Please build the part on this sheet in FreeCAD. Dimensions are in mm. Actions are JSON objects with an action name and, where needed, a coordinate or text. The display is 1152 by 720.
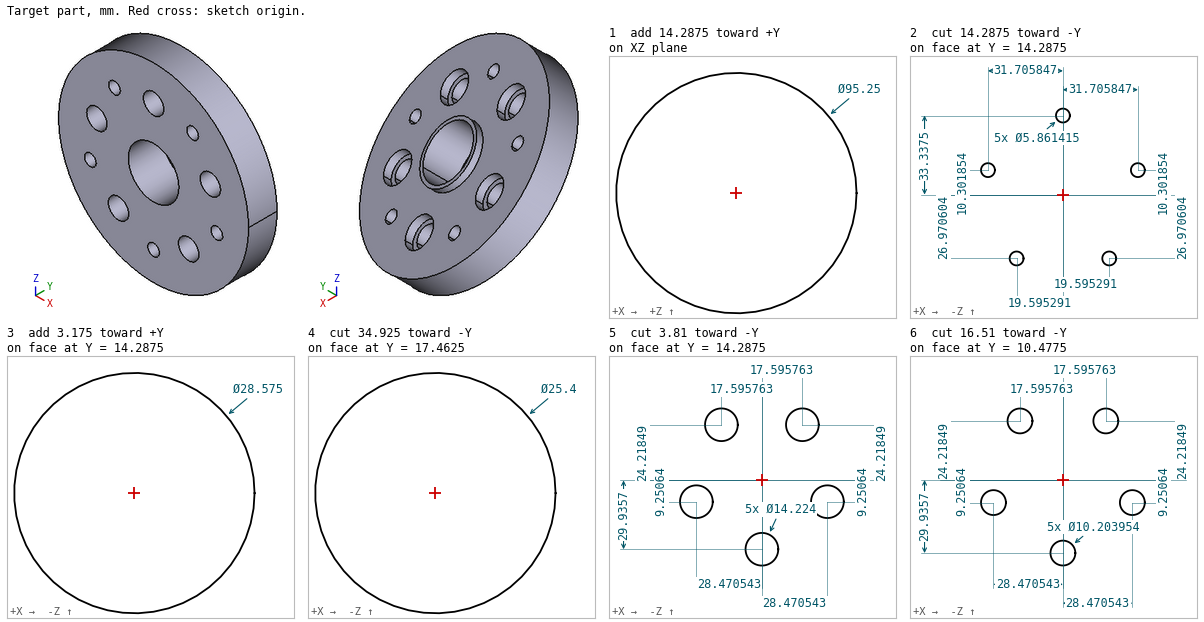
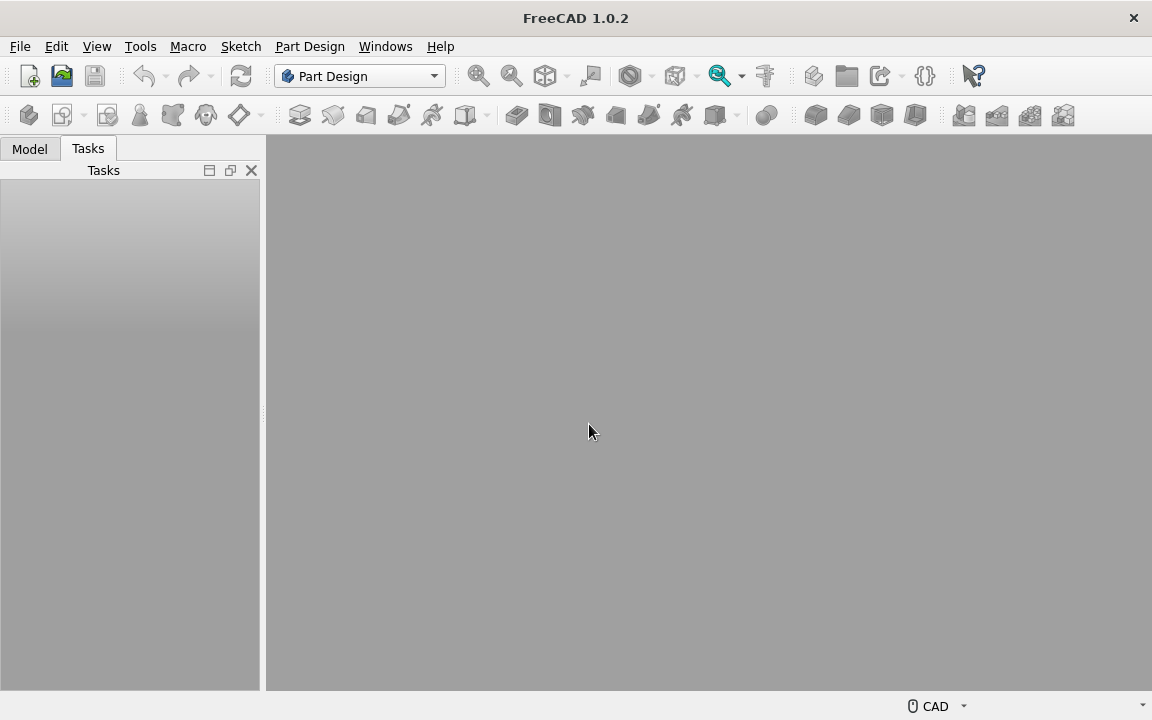
{"action": "left_click", "coordinate": [29, 76]}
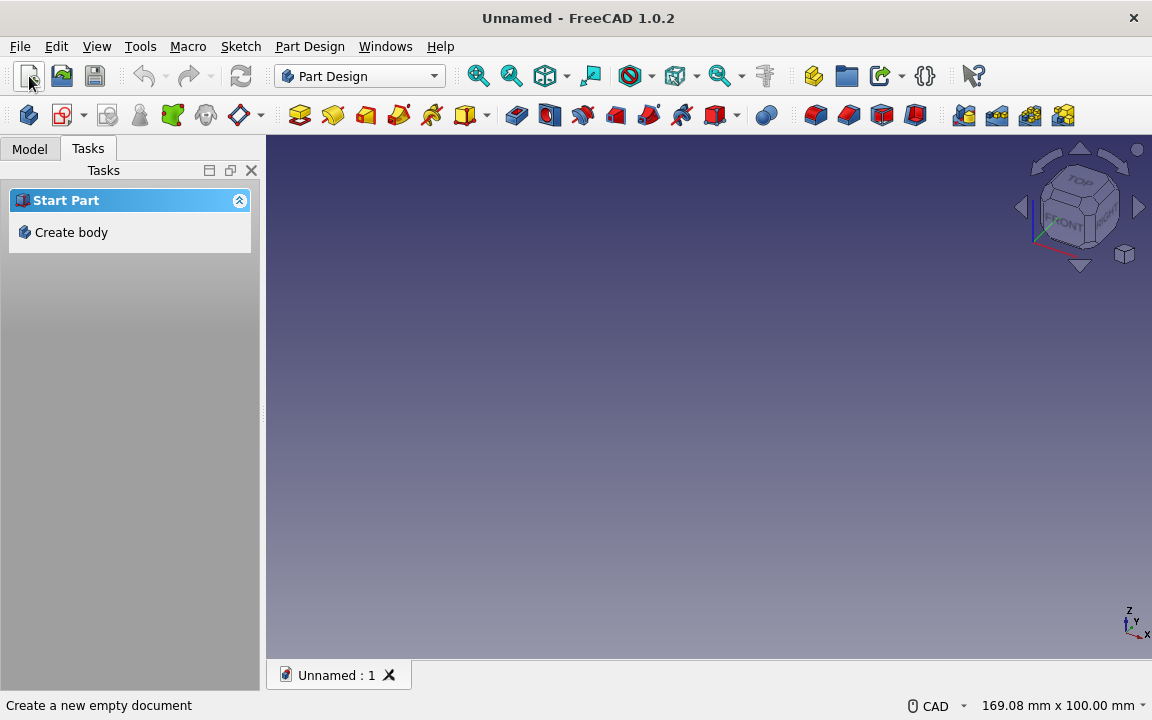
{"action": "left_click", "coordinate": [62, 116]}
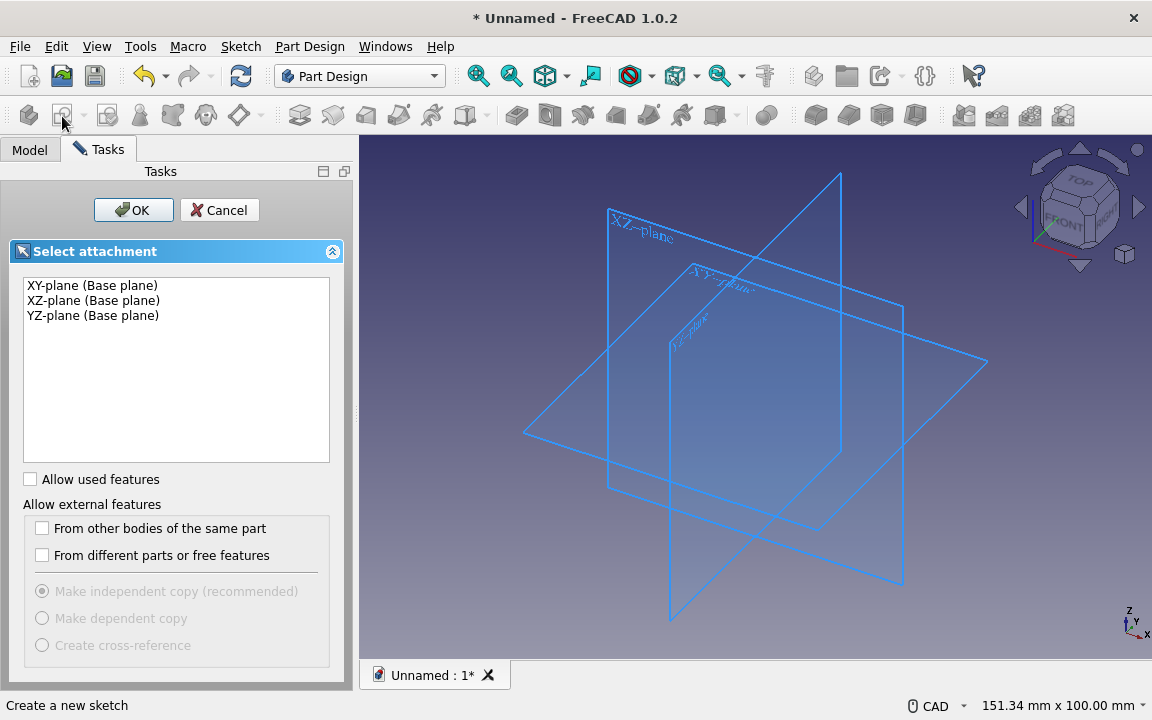
{"action": "left_click", "coordinate": [84, 300]}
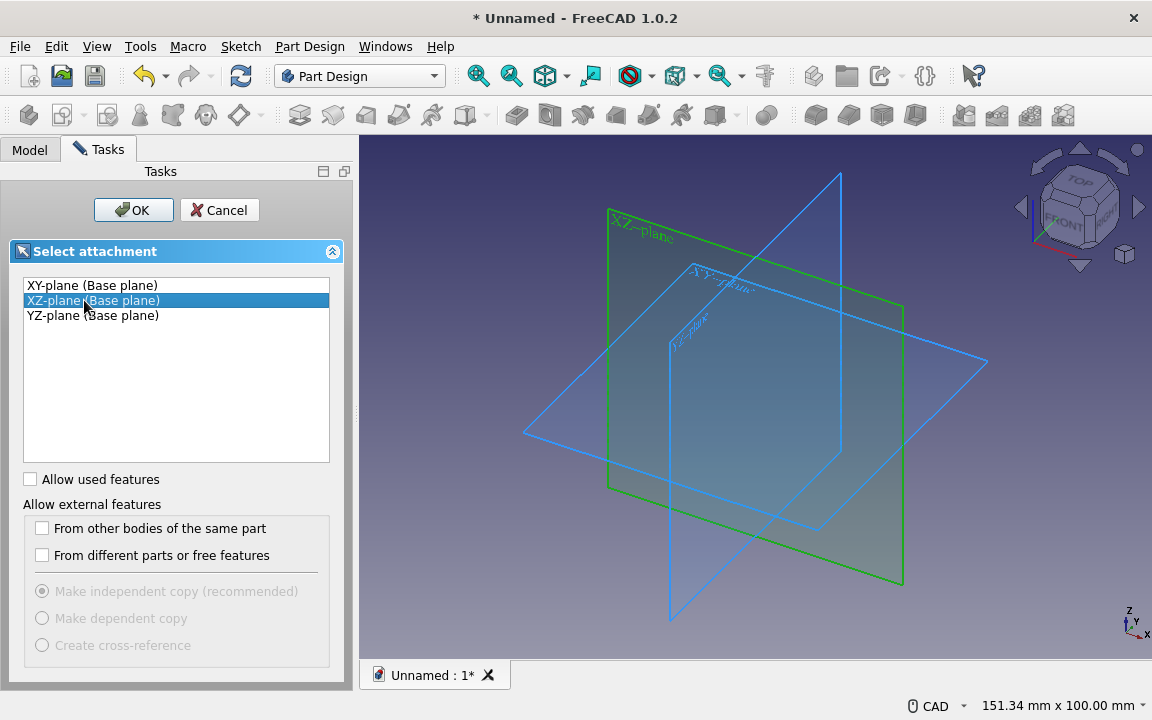
{"action": "left_click", "coordinate": [134, 210]}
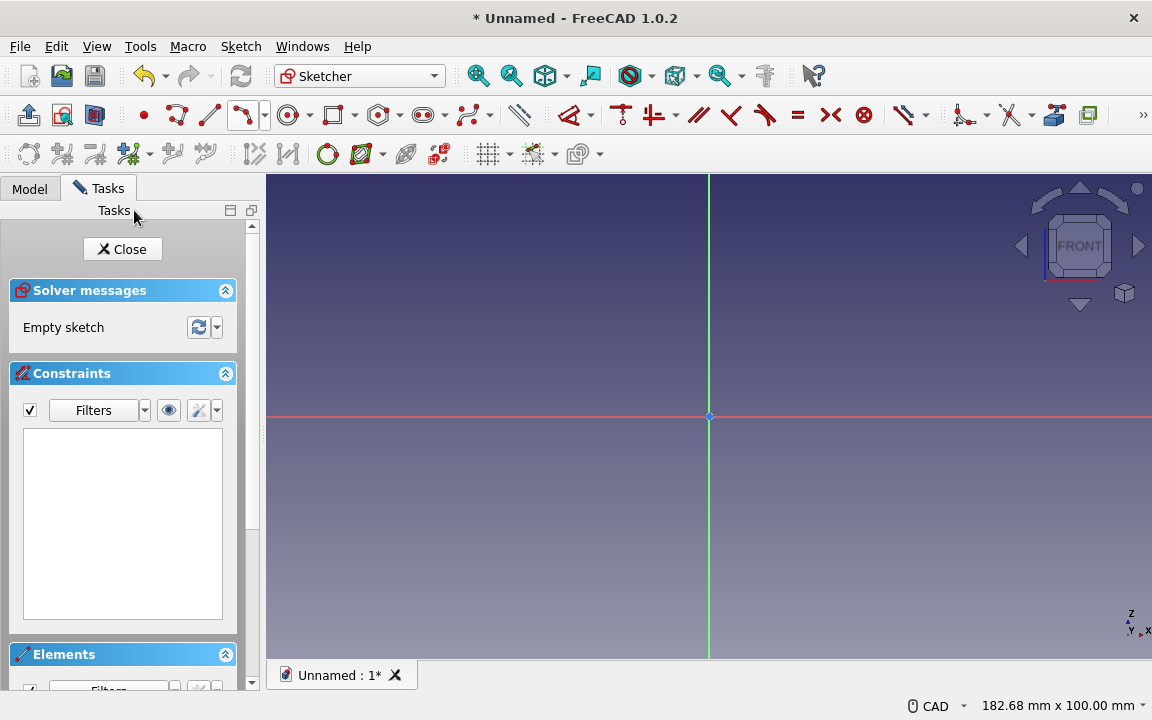
{"action": "scroll", "coordinate": [501, 416], "scroll_direction": "down", "scroll_amount": 2}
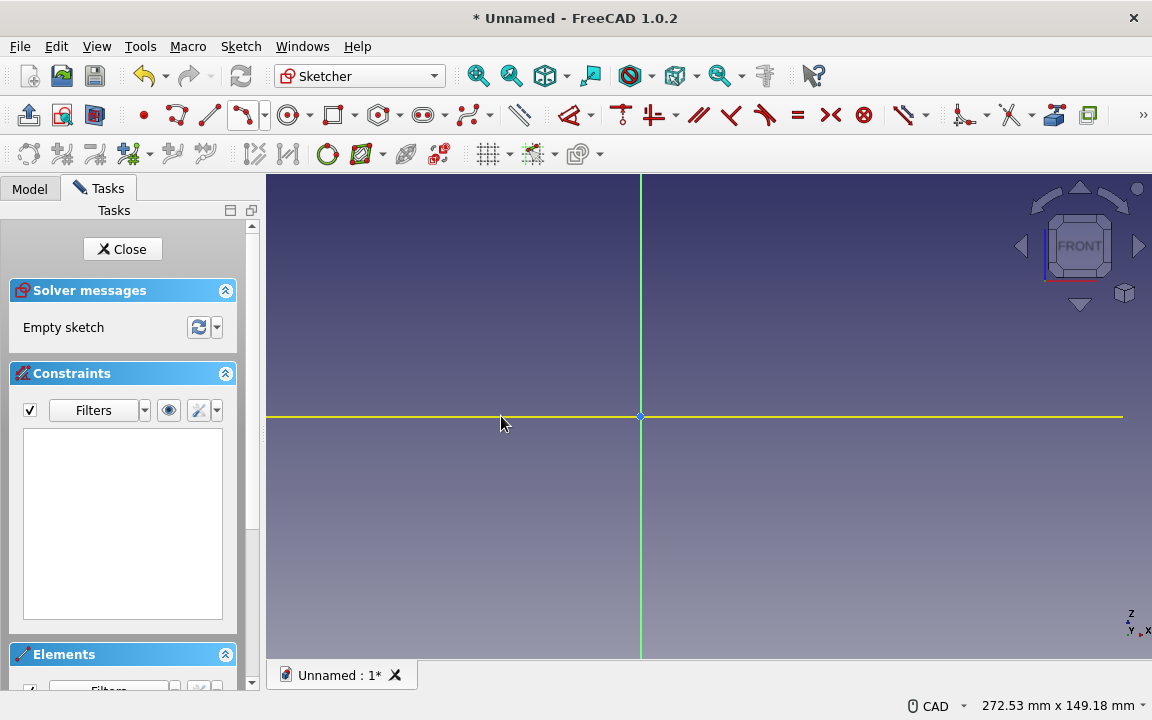
{"action": "left_click", "coordinate": [288, 116]}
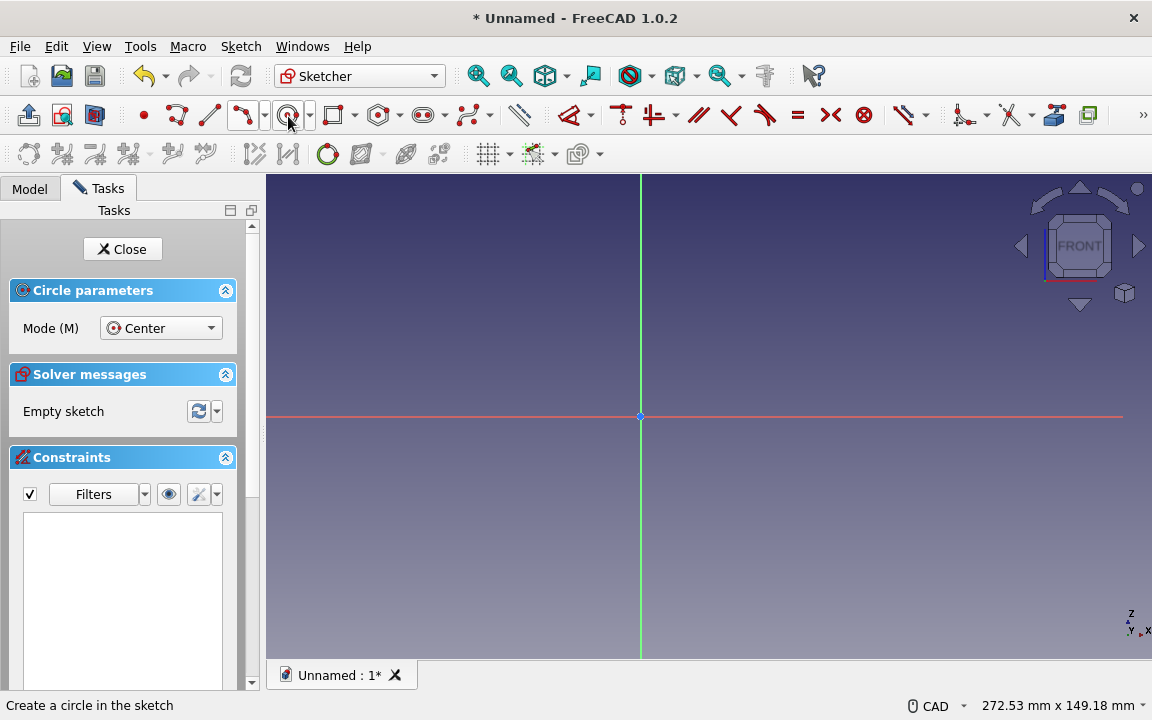
{"action": "left_click", "coordinate": [641, 416]}
{"action": "mouse_move", "coordinate": [750, 307]}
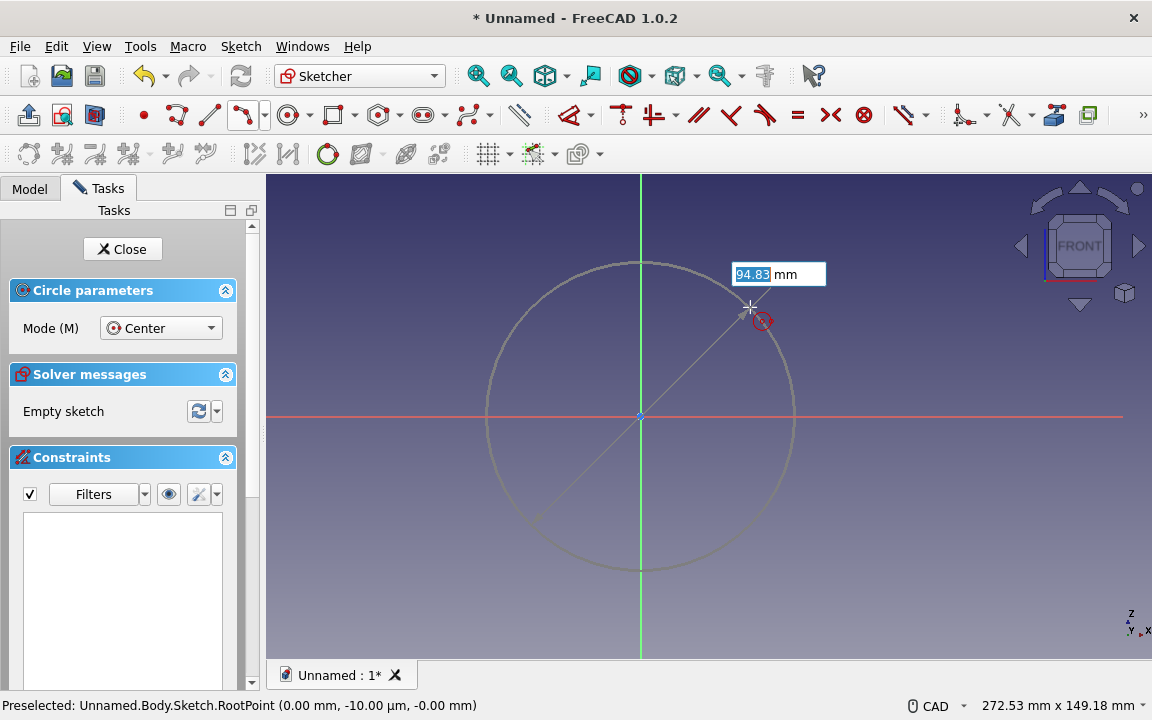
{"action": "type", "text": "95.25"}
{"action": "key", "text": "Return"}
{"action": "key", "text": "Escape"}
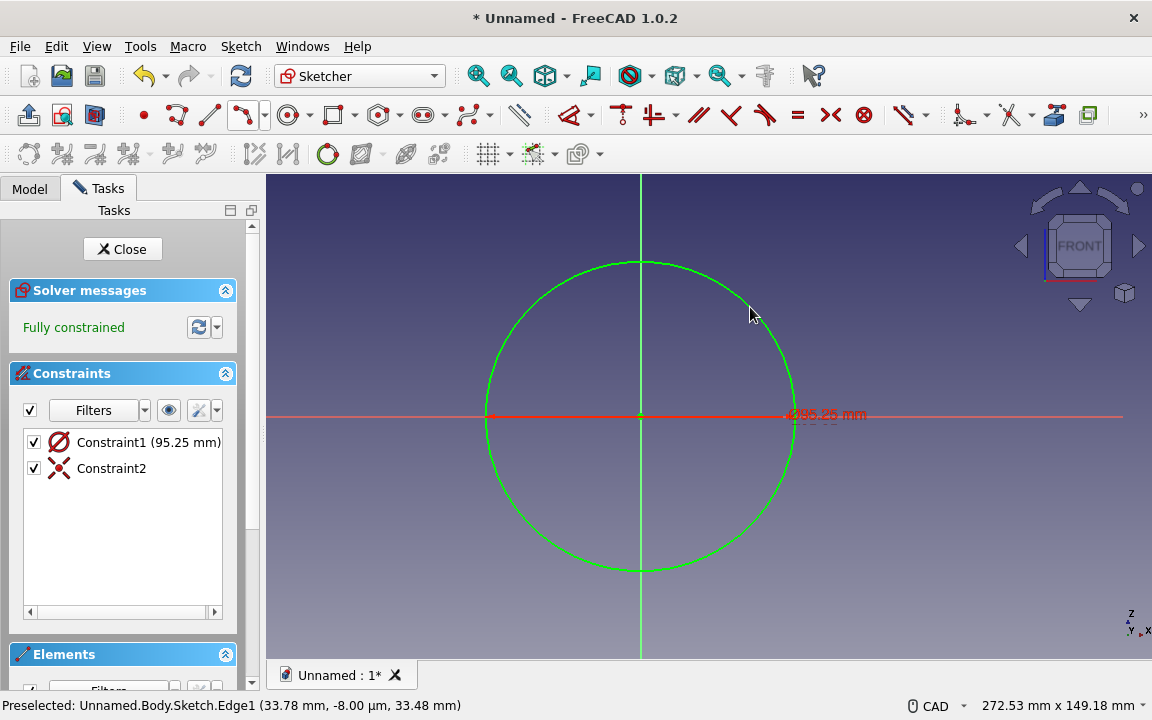
{"action": "left_click", "coordinate": [123, 249]}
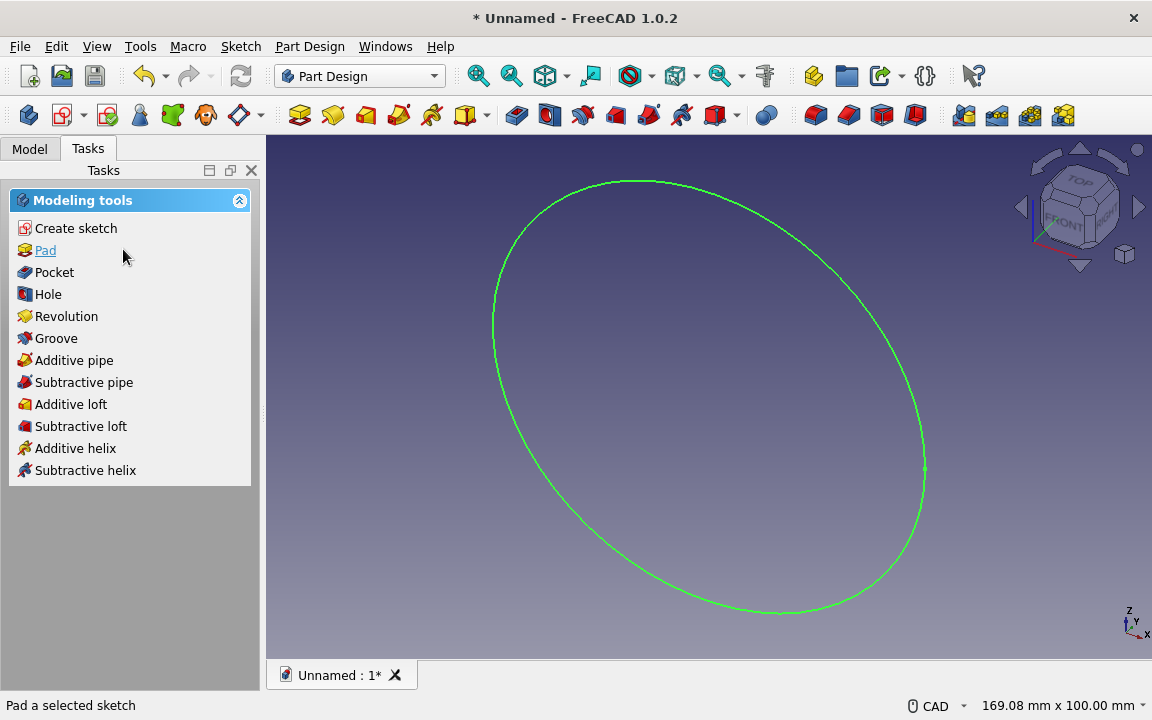
{"action": "left_click", "coordinate": [300, 116]}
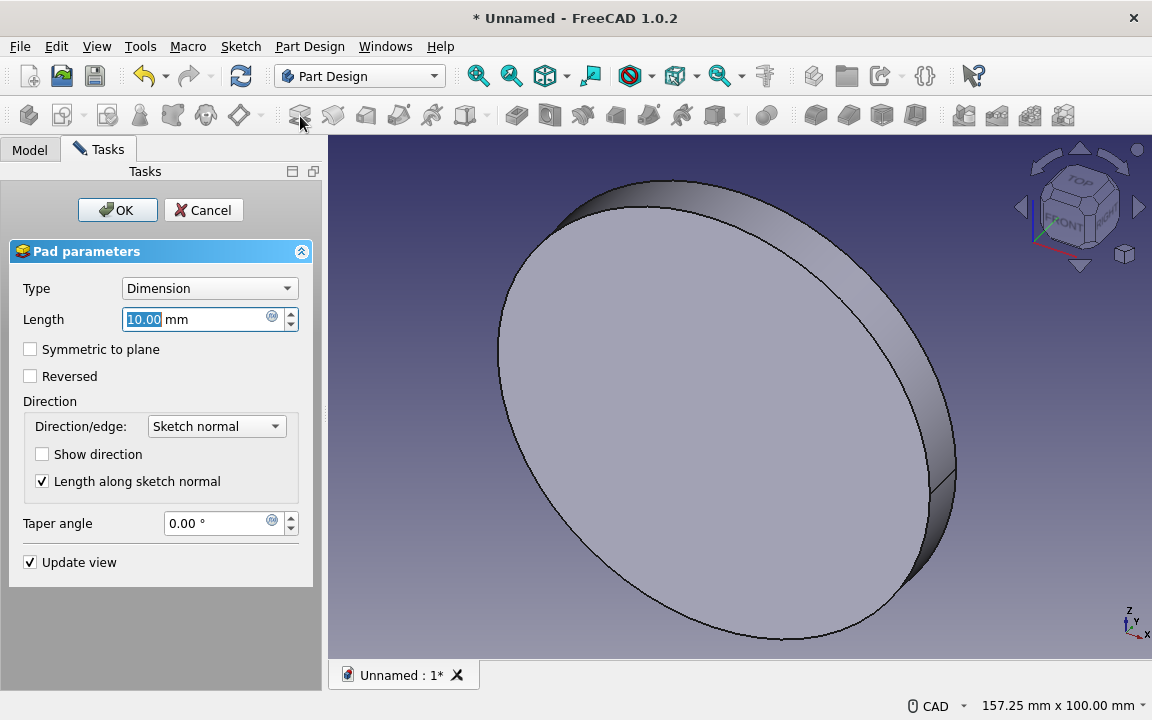
{"action": "type", "text": "14.2875"}
{"action": "key", "text": "Tab"}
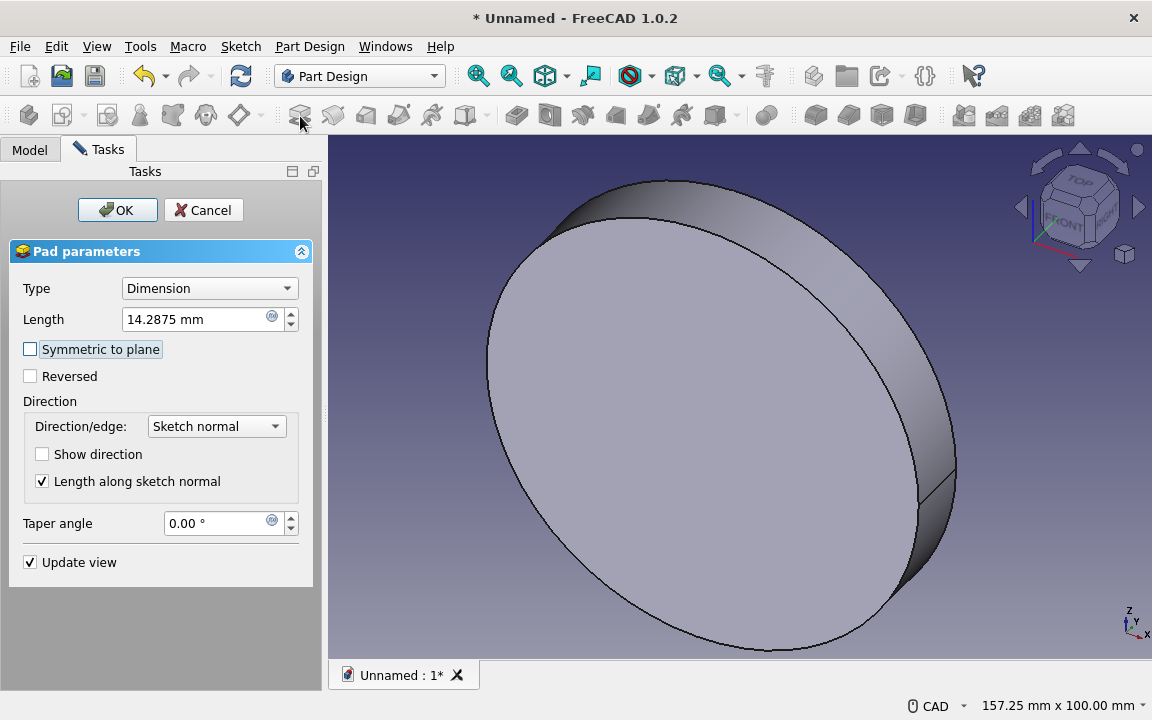
{"action": "left_click", "coordinate": [31, 376]}